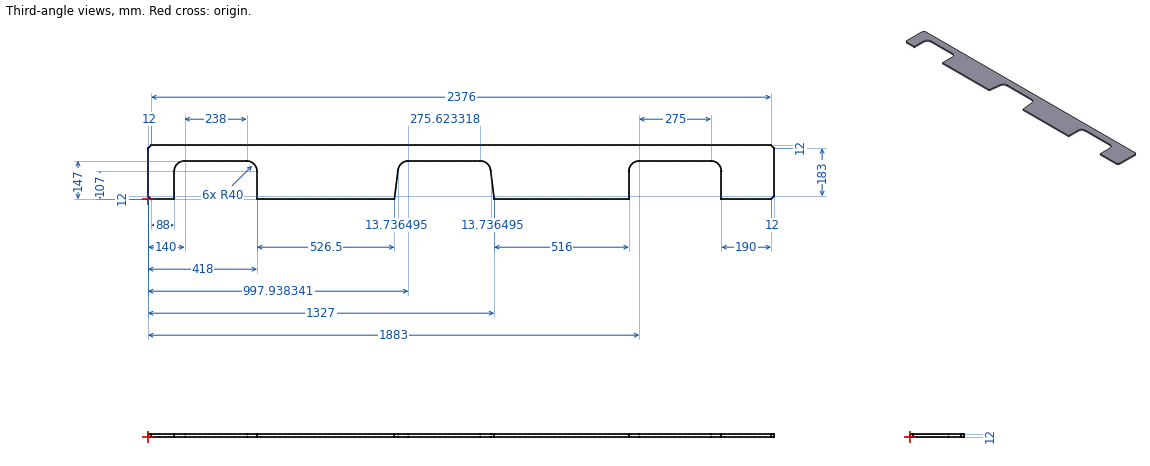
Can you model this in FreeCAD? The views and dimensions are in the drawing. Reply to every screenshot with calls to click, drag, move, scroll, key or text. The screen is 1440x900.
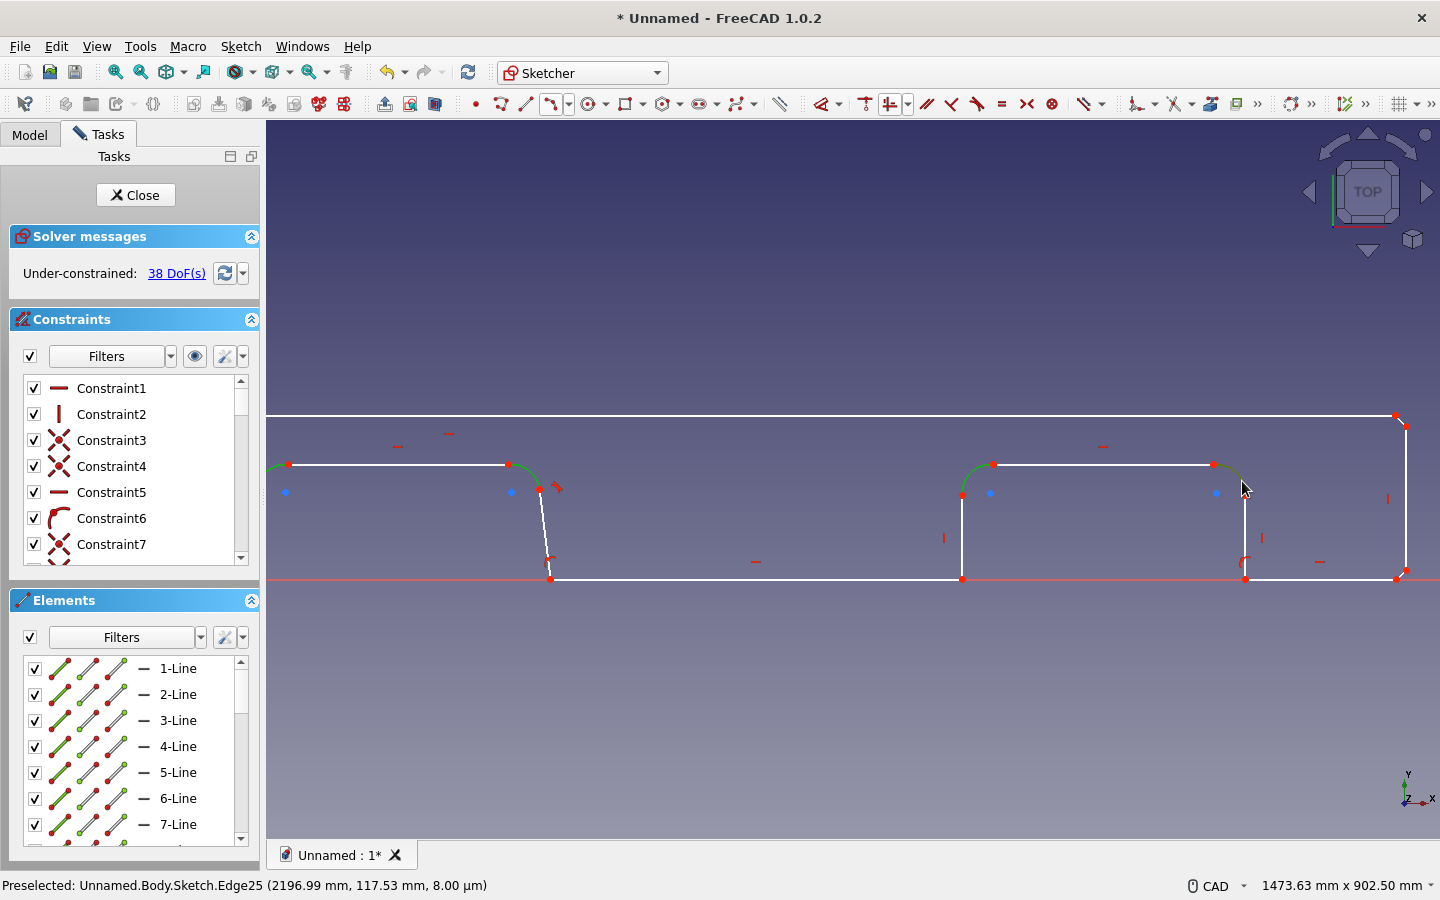
scroll(979, 469, down, 5)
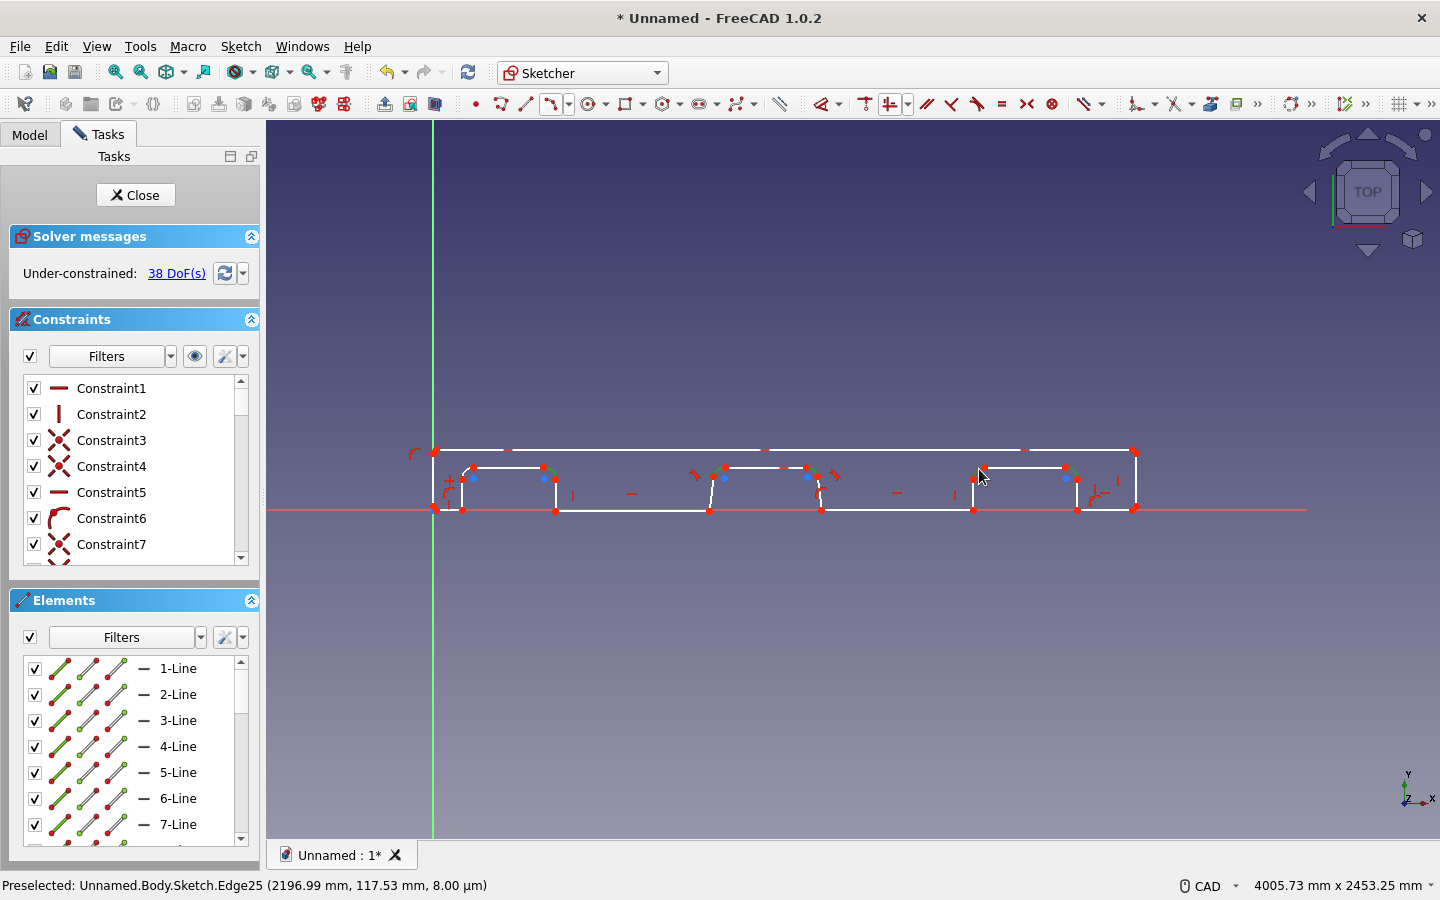
scroll(468, 469, up, 5)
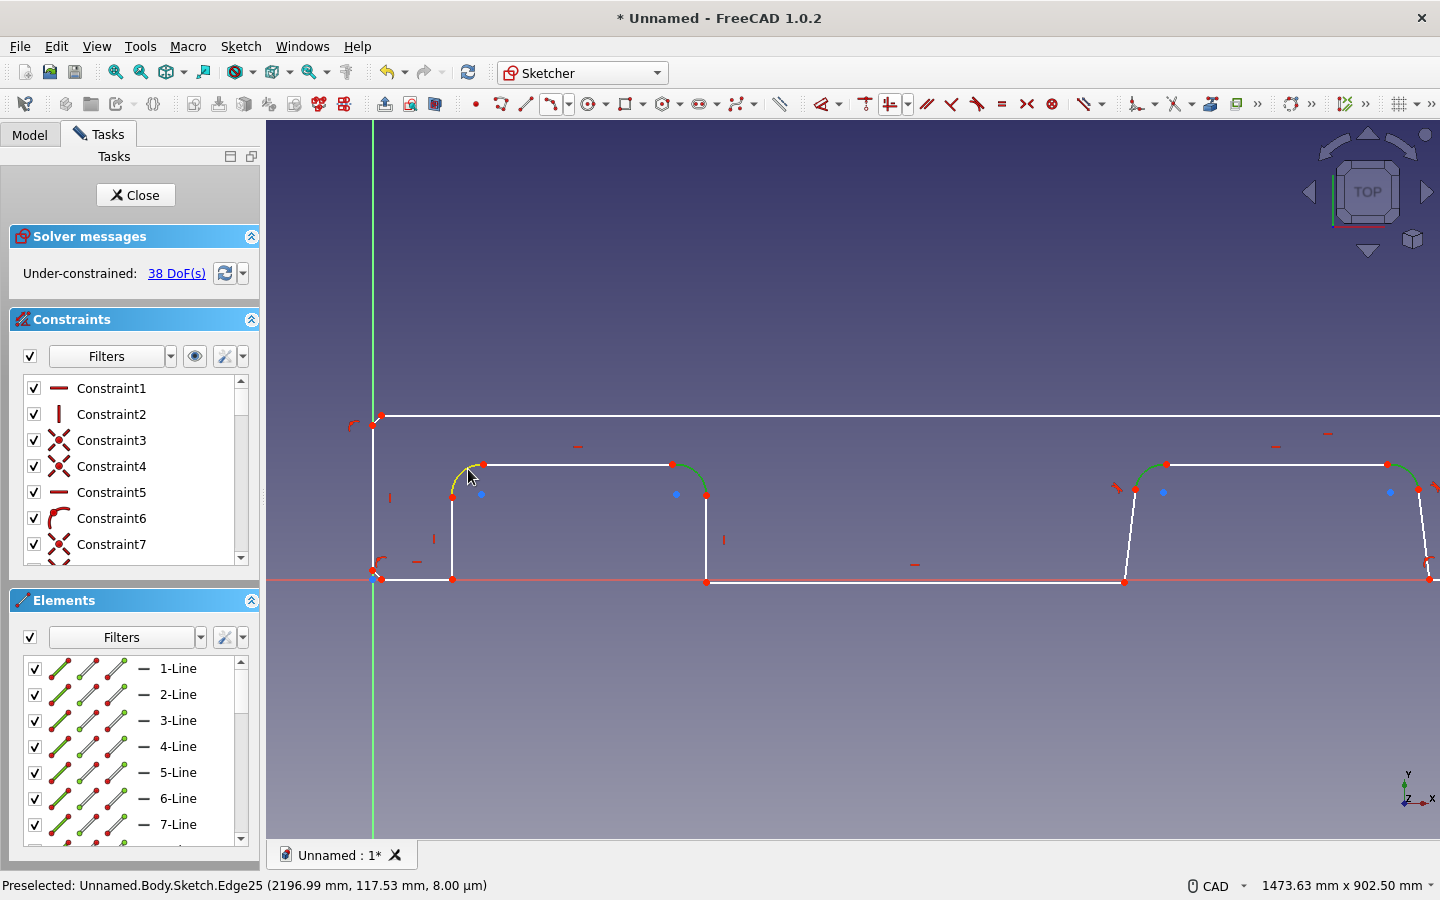
click(469, 468)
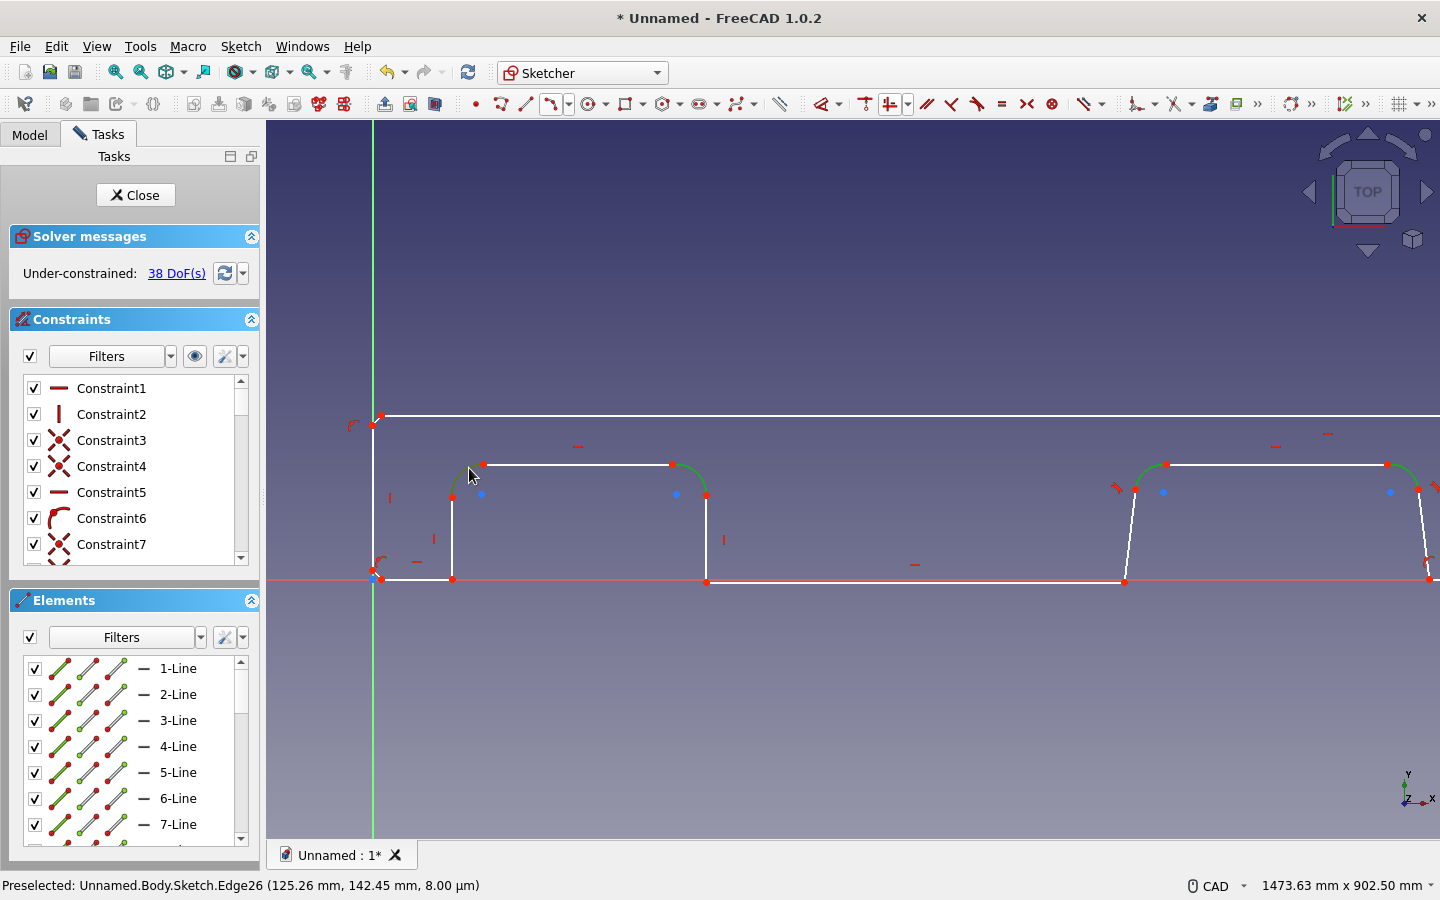
click(1002, 104)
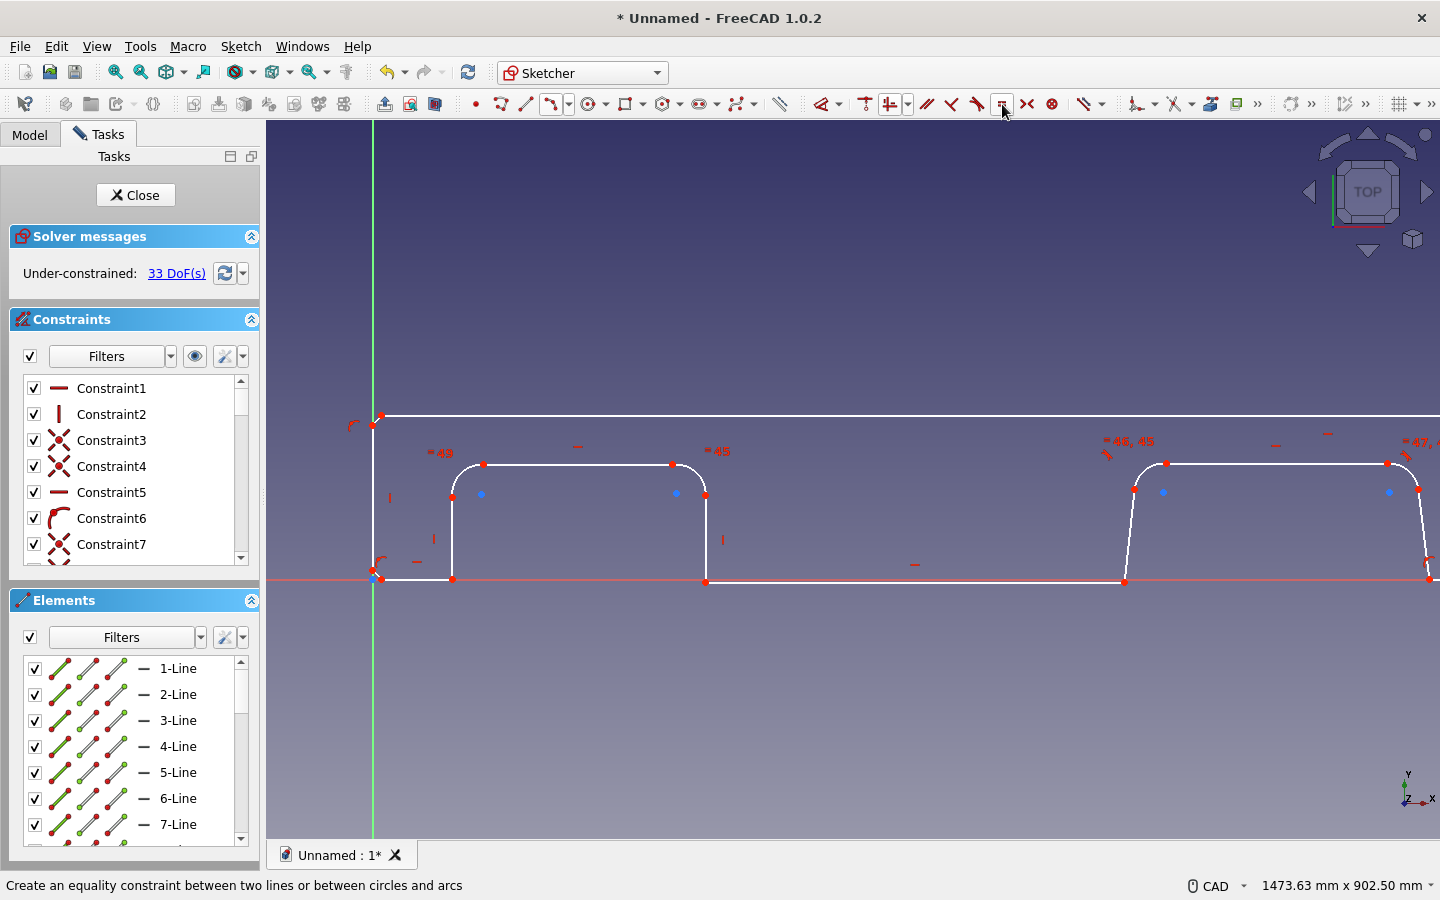
click(820, 104)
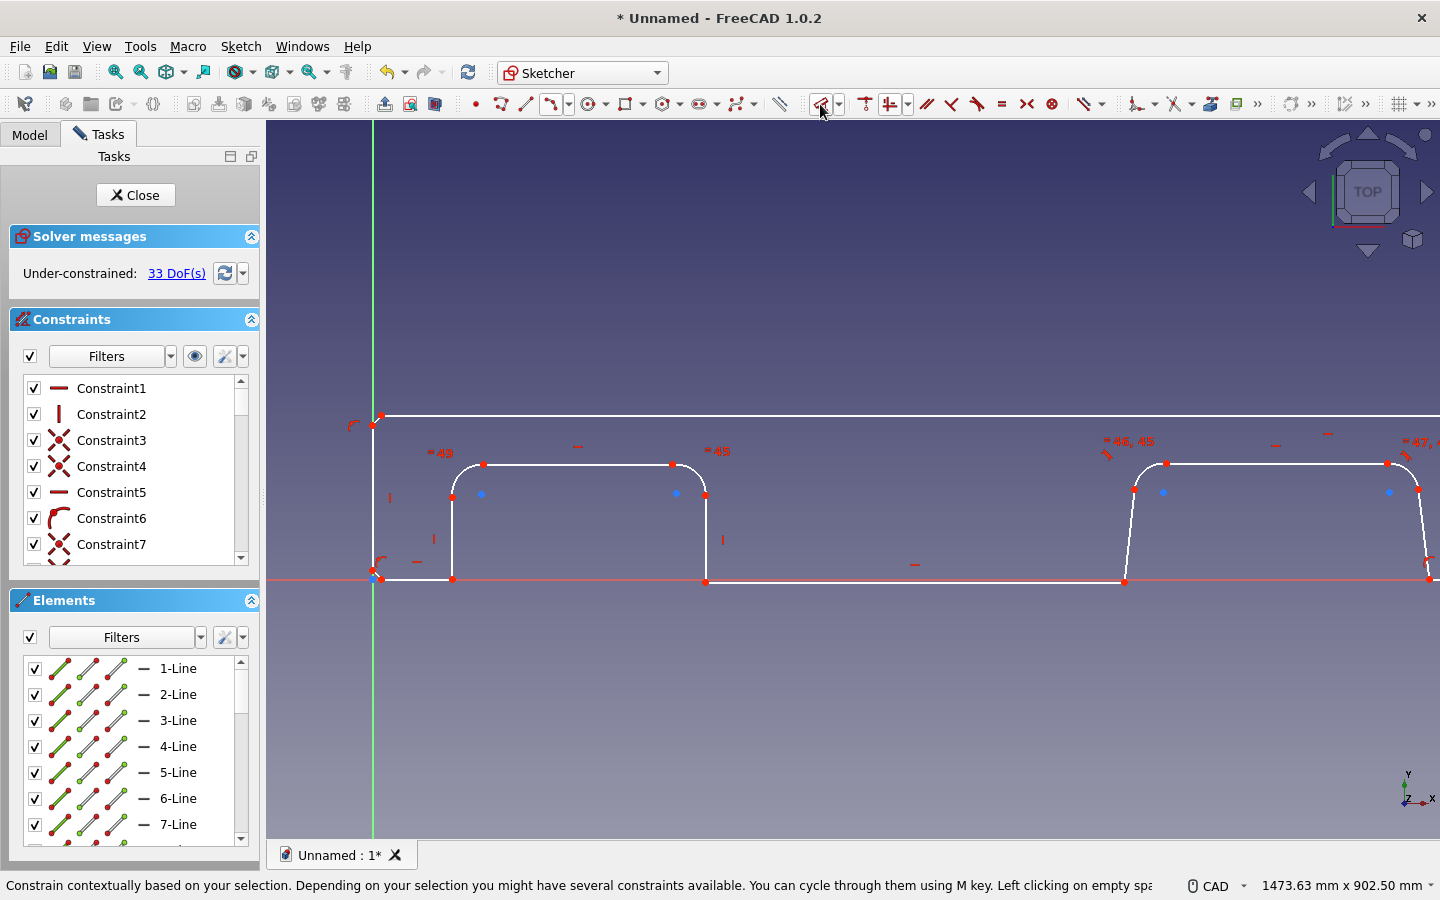
scroll(703, 481, up, 2)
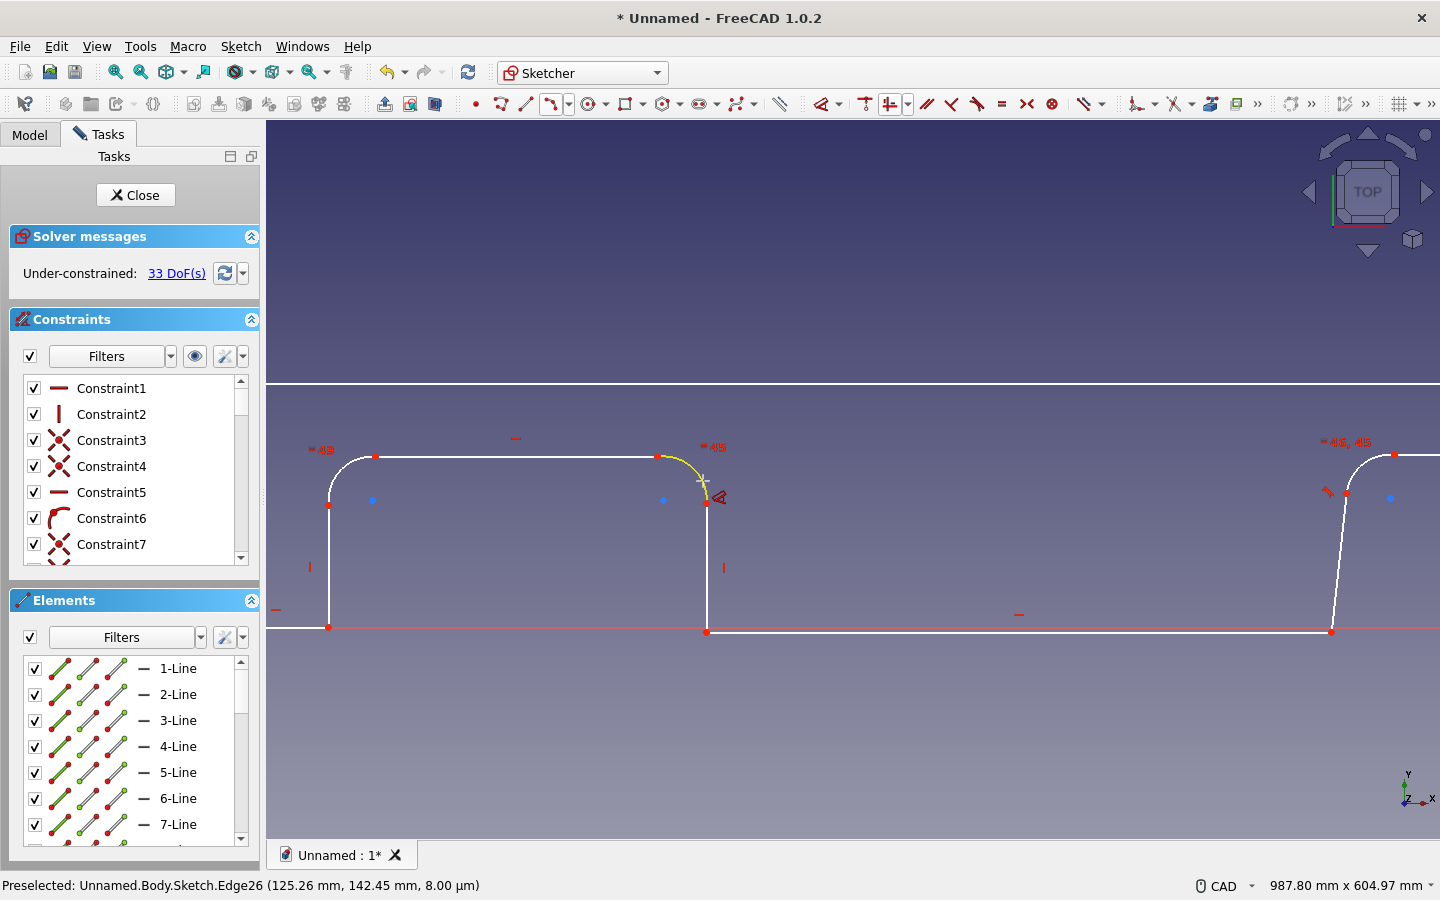
click(702, 481)
click(731, 467)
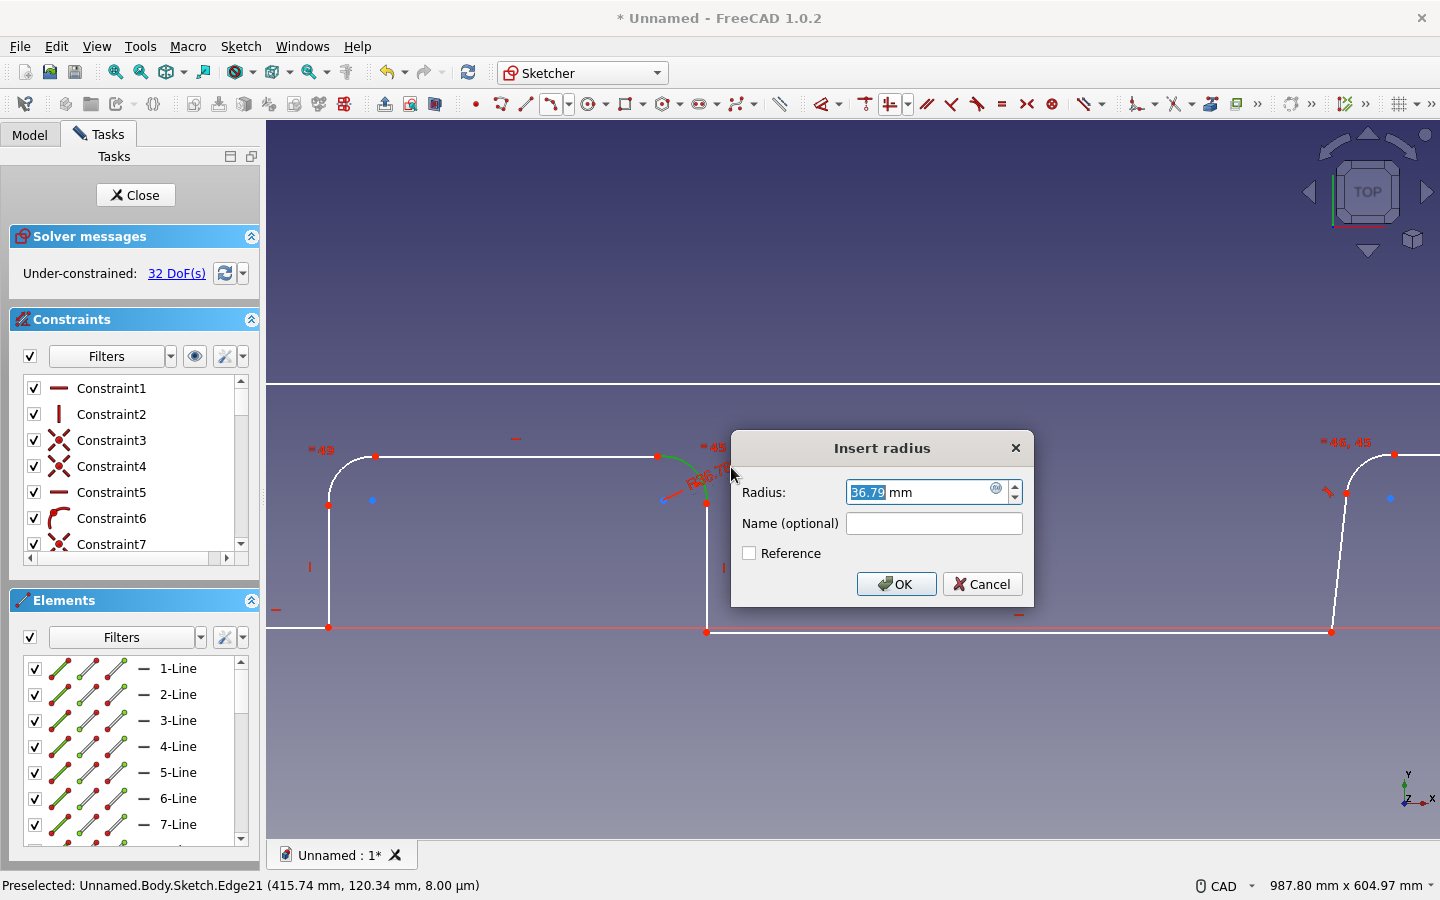
text(40)
key(Return)
key(Escape)